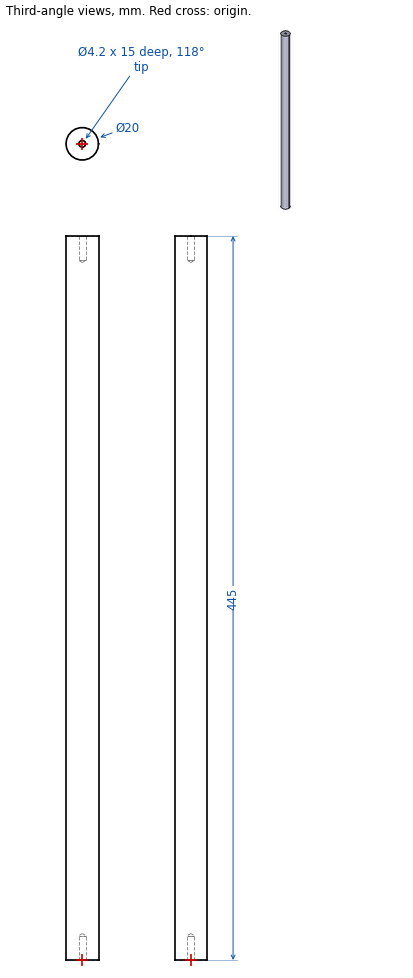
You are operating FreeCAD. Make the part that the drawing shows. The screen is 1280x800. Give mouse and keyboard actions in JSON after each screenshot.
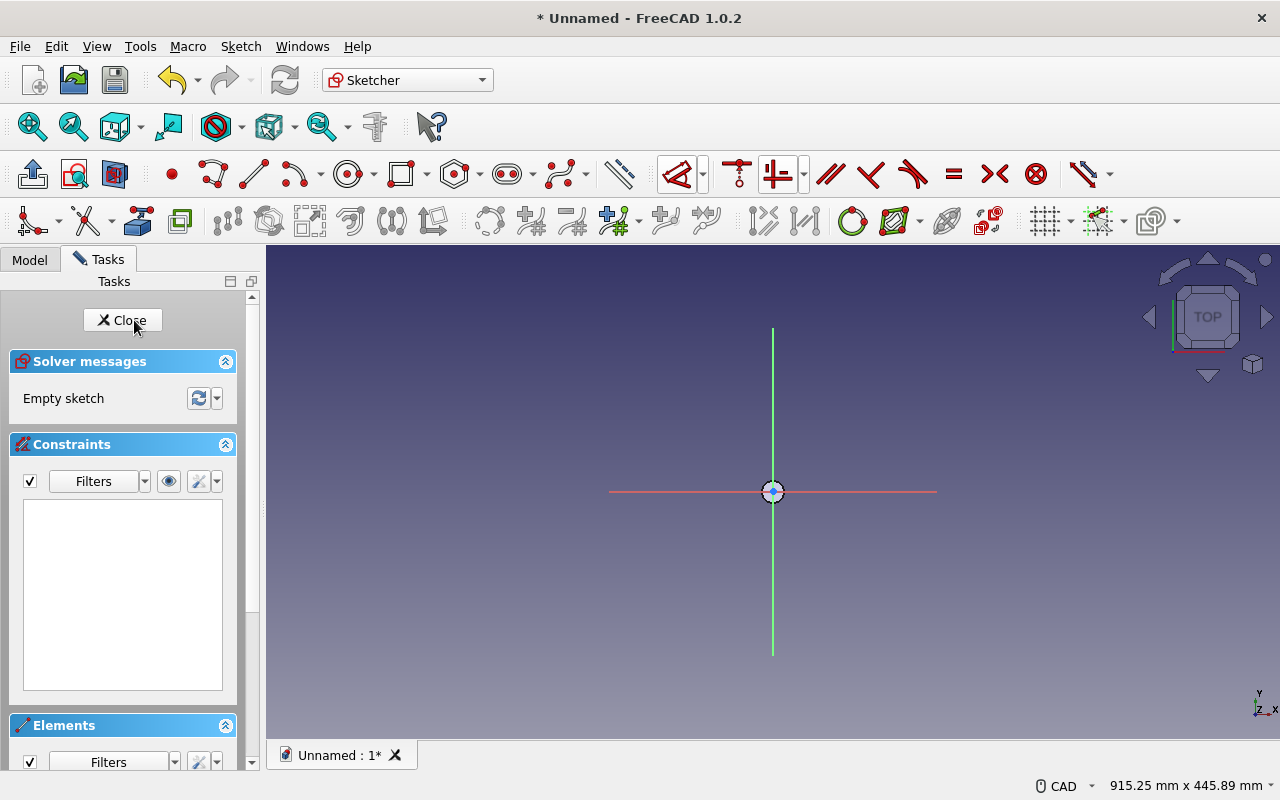
{"action": "scroll", "coordinate": [777, 492], "scroll_direction": "up", "scroll_amount": 15}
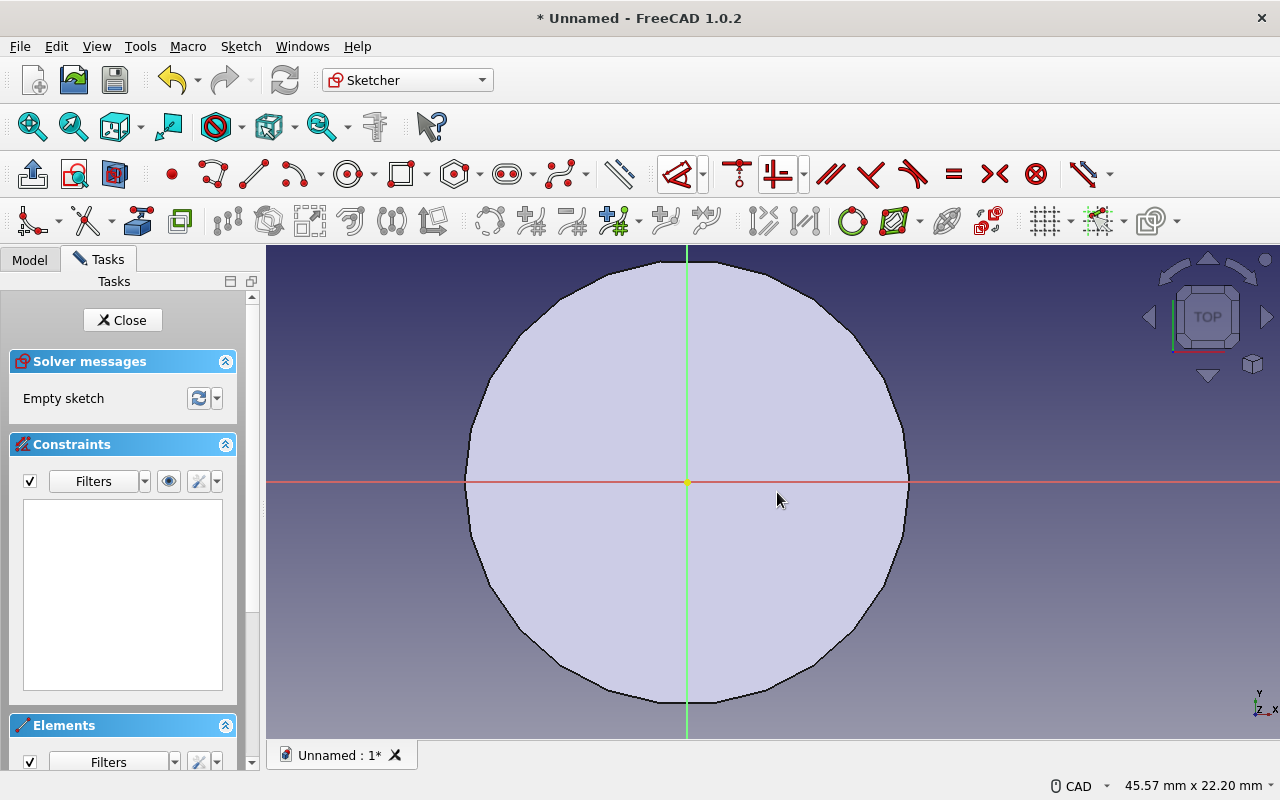
{"action": "scroll", "coordinate": [680, 478], "scroll_direction": "up", "scroll_amount": 6}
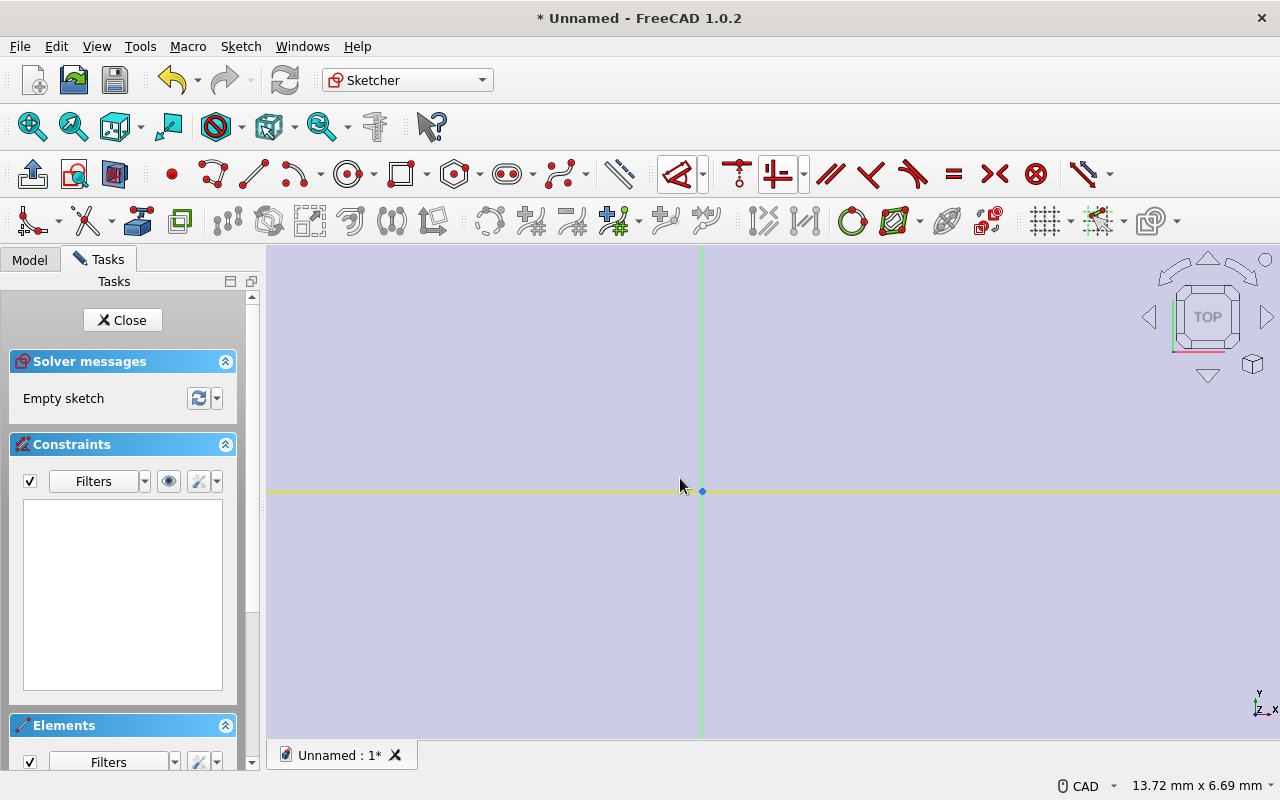
{"action": "key", "text": "g c"}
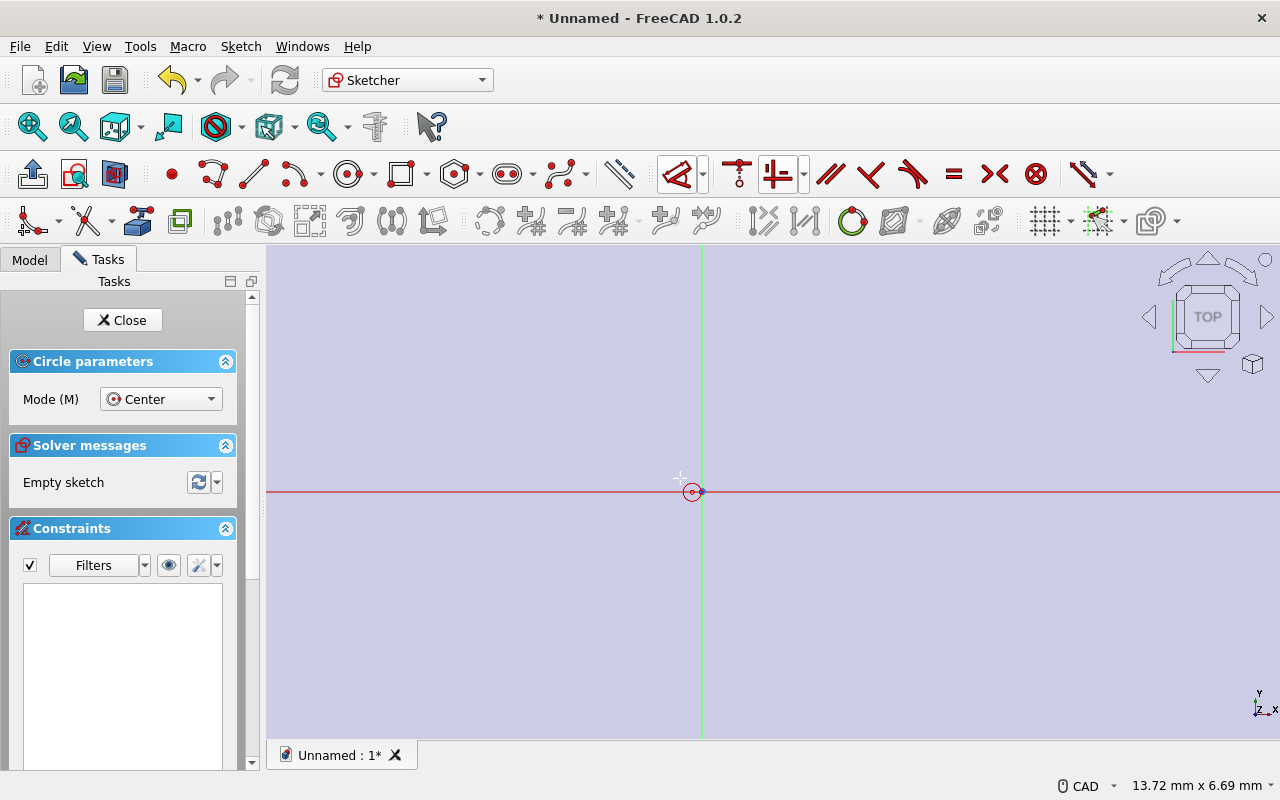
{"action": "left_click", "coordinate": [702, 492]}
{"action": "left_click", "coordinate": [812, 382]}
{"action": "key", "text": "Escape"}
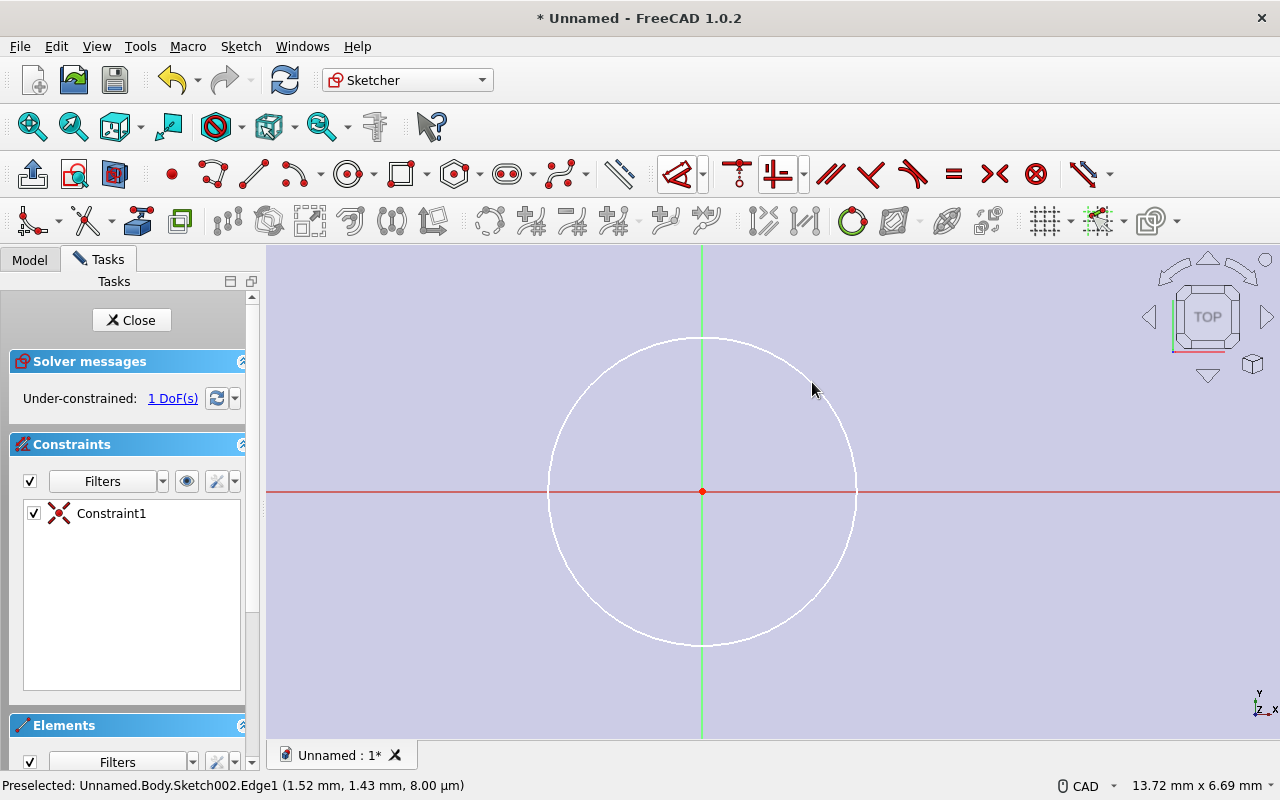
{"action": "left_click", "coordinate": [811, 382]}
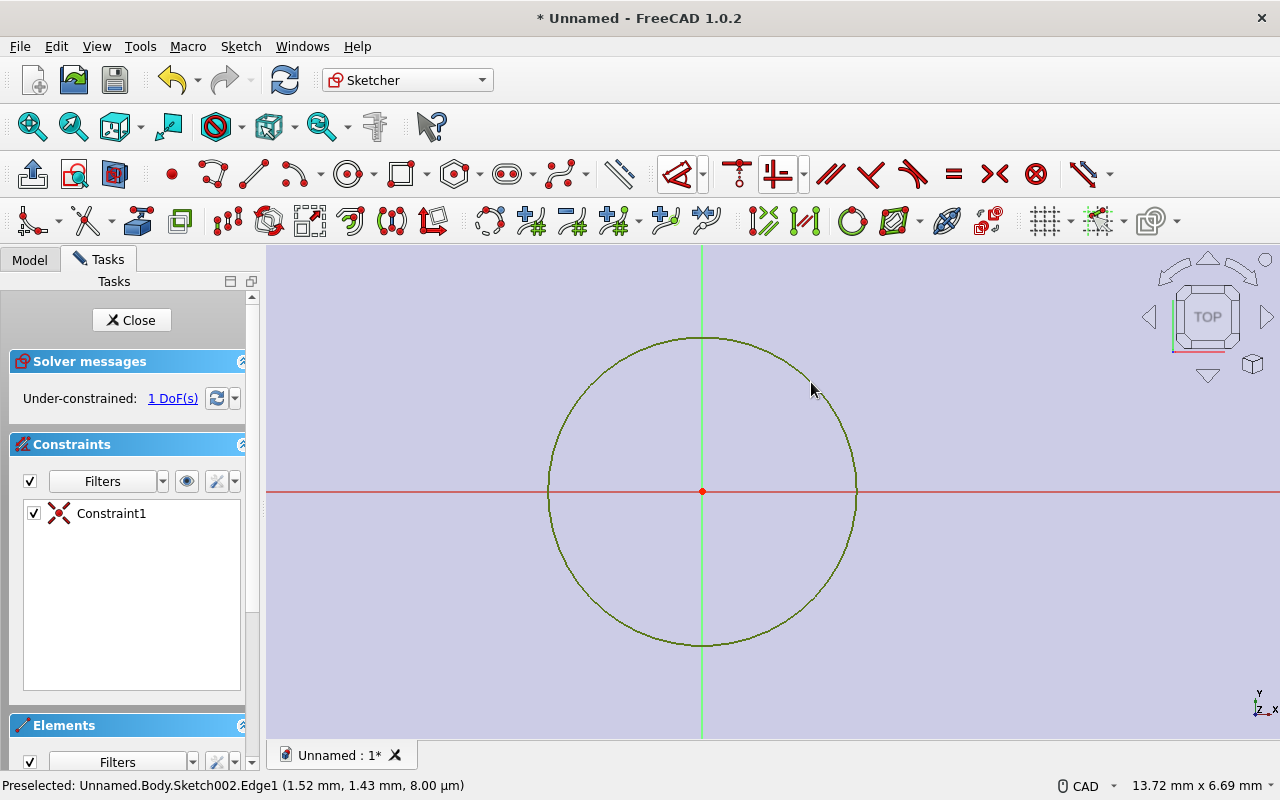
{"action": "left_click", "coordinate": [702, 174]}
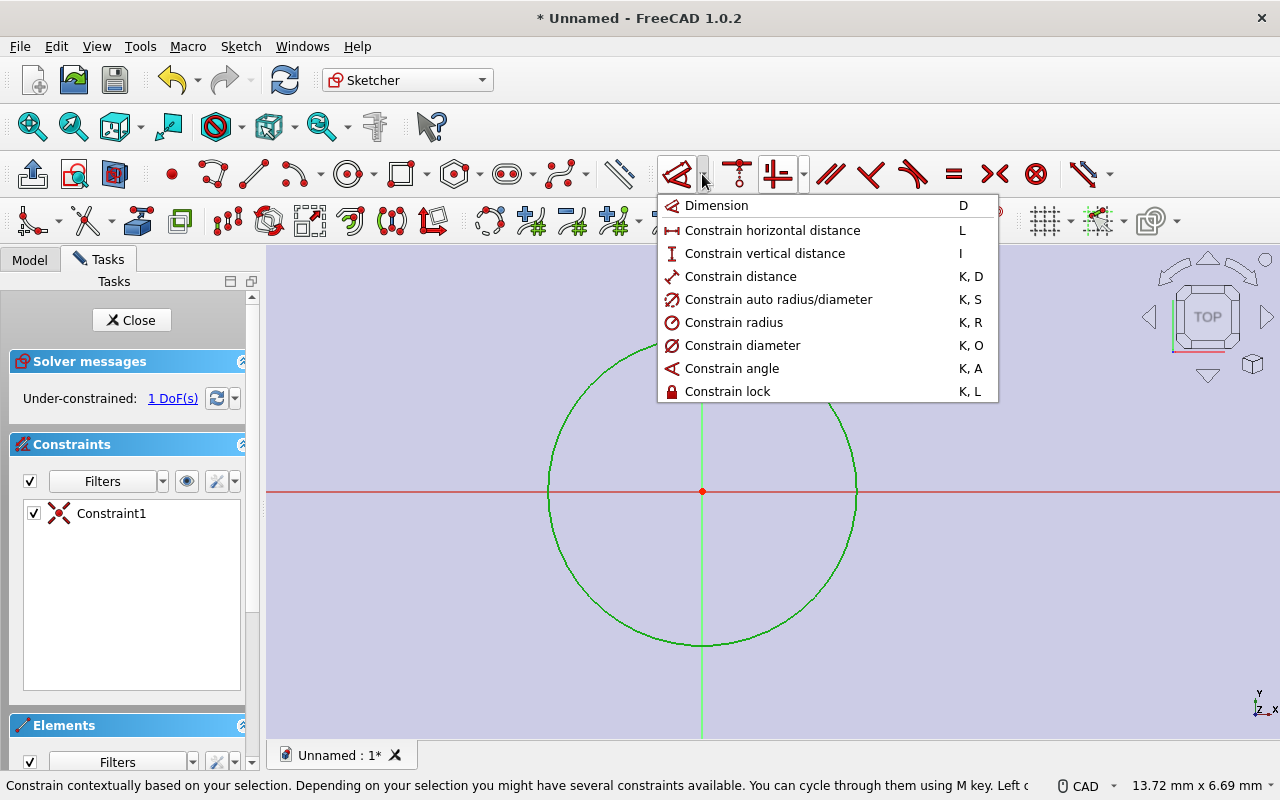
{"action": "left_click", "coordinate": [828, 346]}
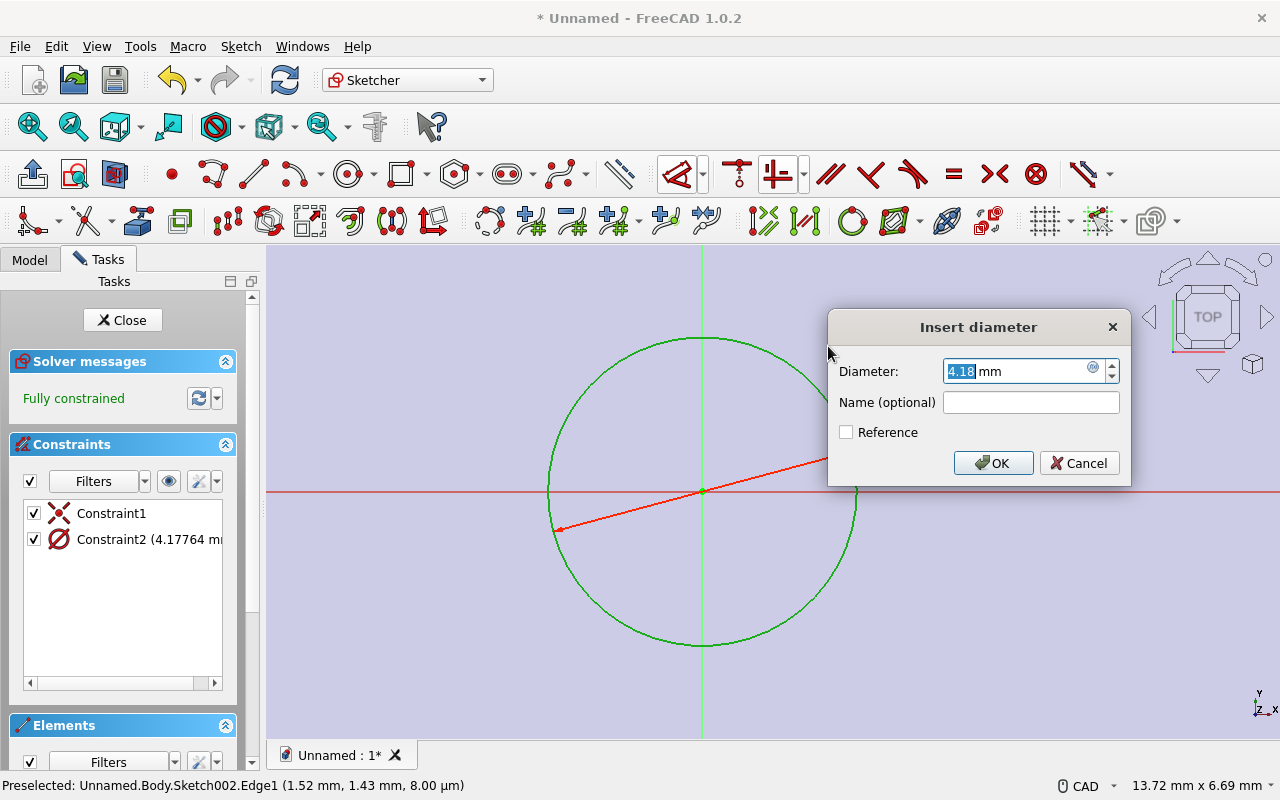
{"action": "type", "text": "4.2"}
{"action": "key", "text": "Return"}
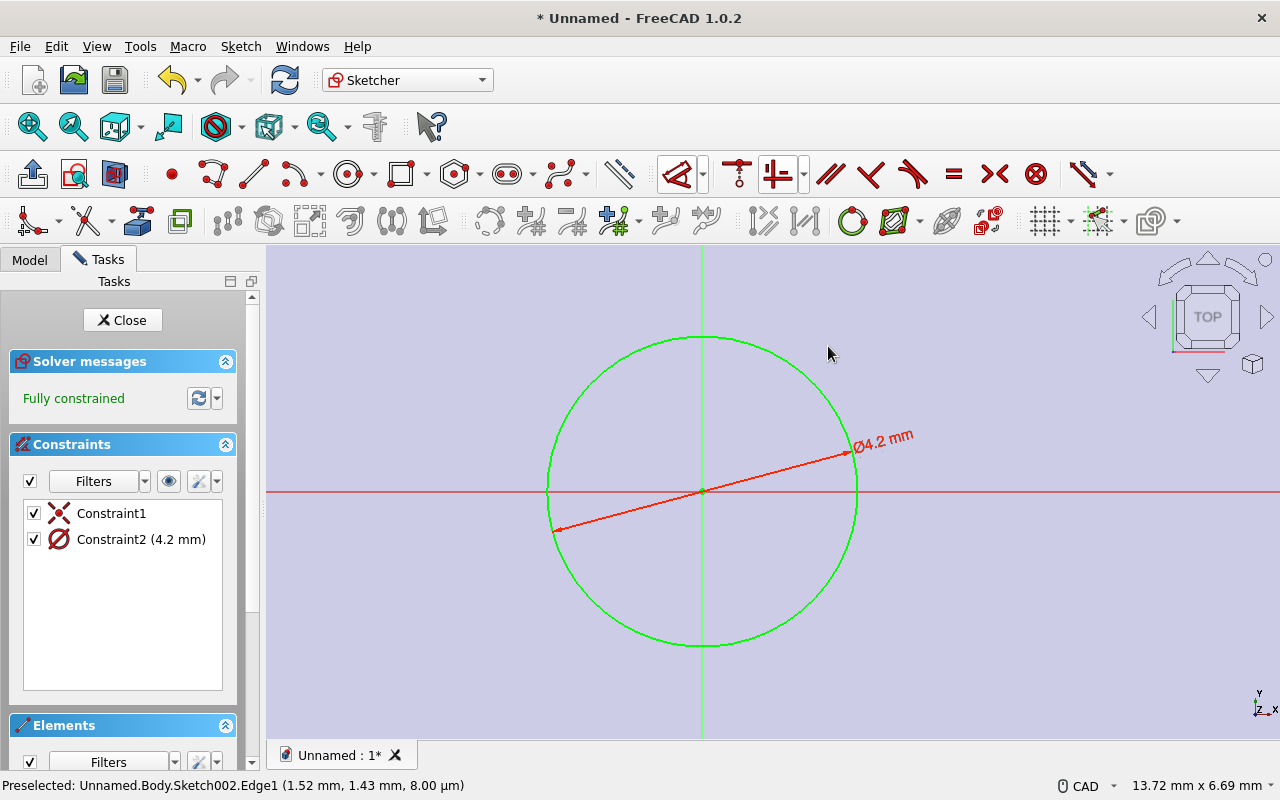
{"action": "left_click", "coordinate": [123, 320]}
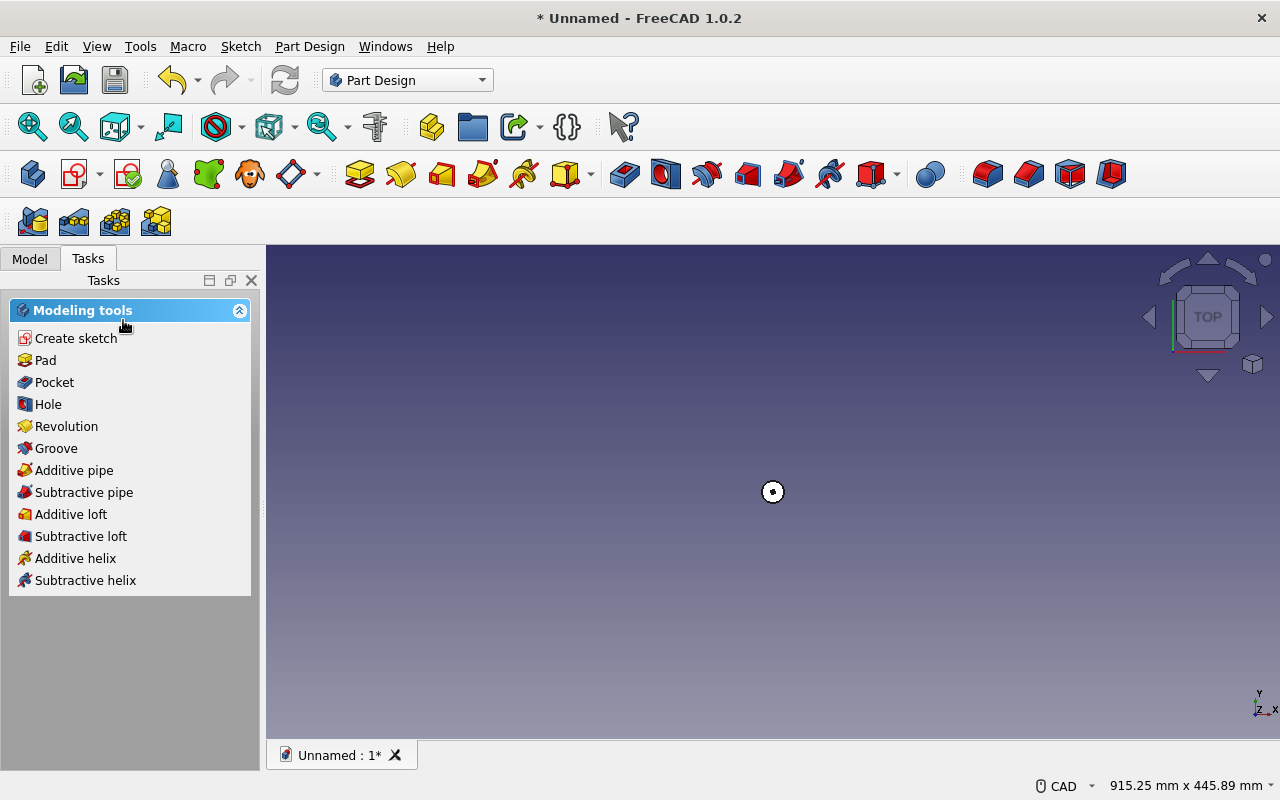
{"action": "left_click", "coordinate": [666, 174]}